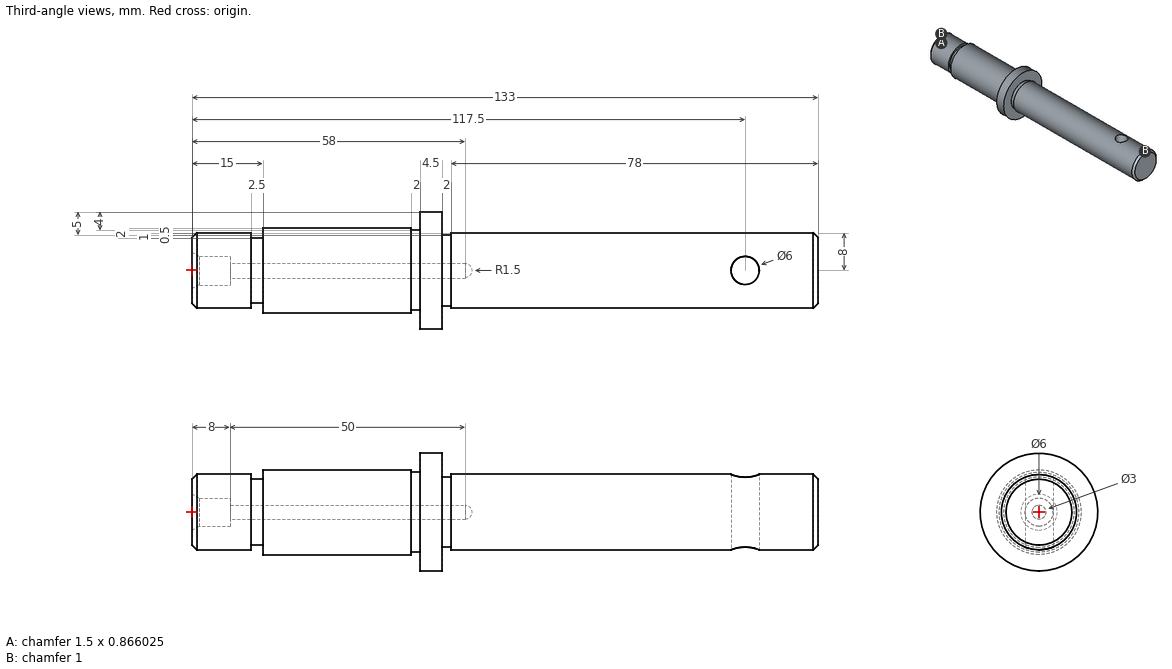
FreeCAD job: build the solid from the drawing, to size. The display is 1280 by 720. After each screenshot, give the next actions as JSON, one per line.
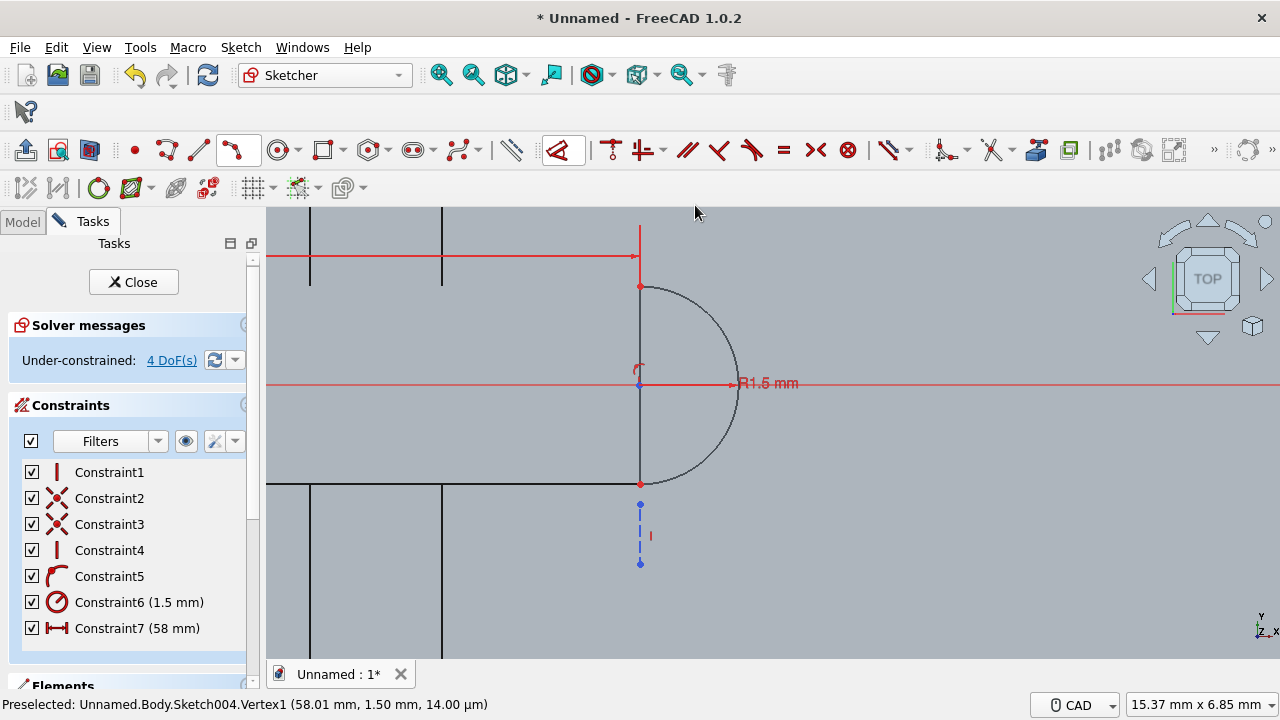
{"action": "left_click", "coordinate": [640, 505]}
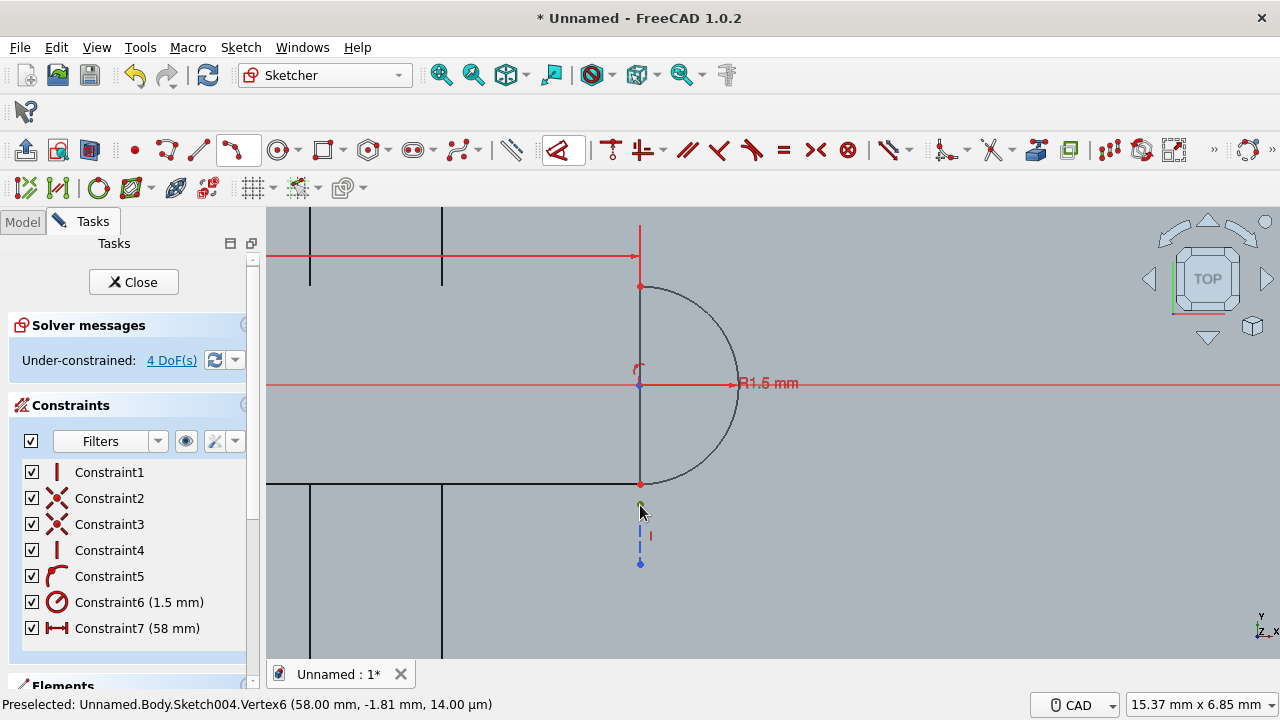
{"action": "left_click", "coordinate": [580, 150]}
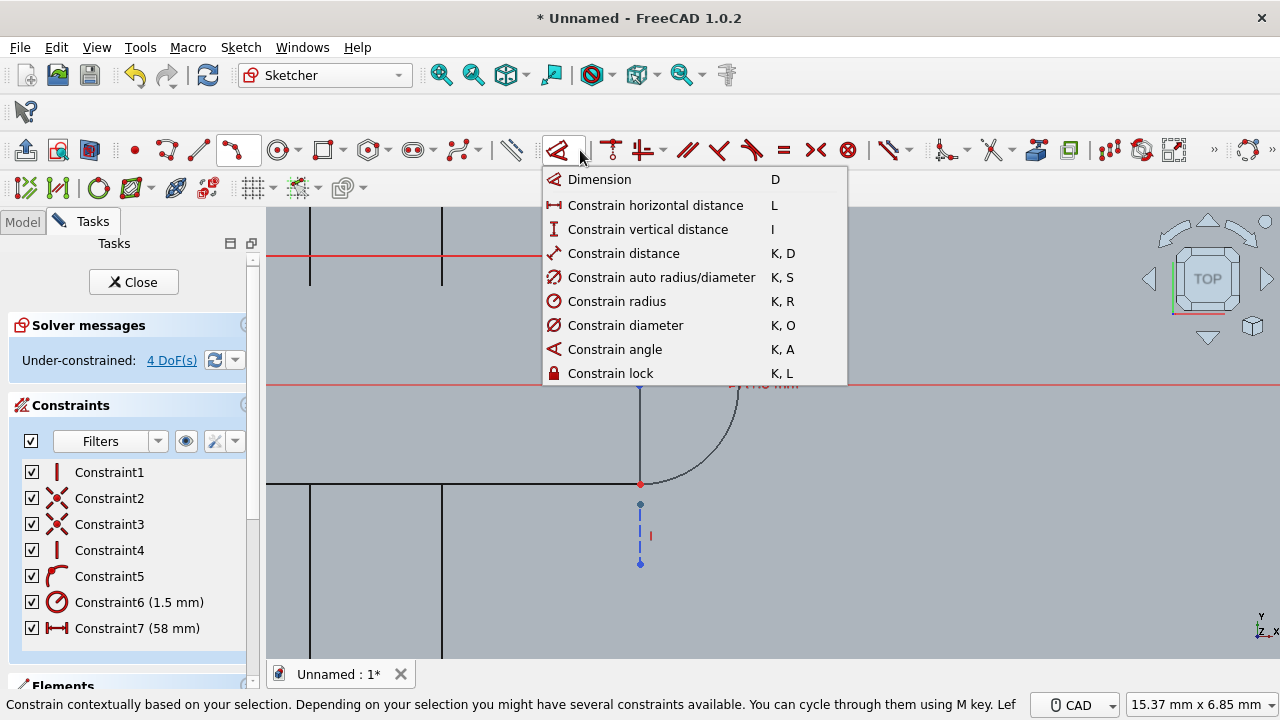
{"action": "left_click", "coordinate": [695, 205]}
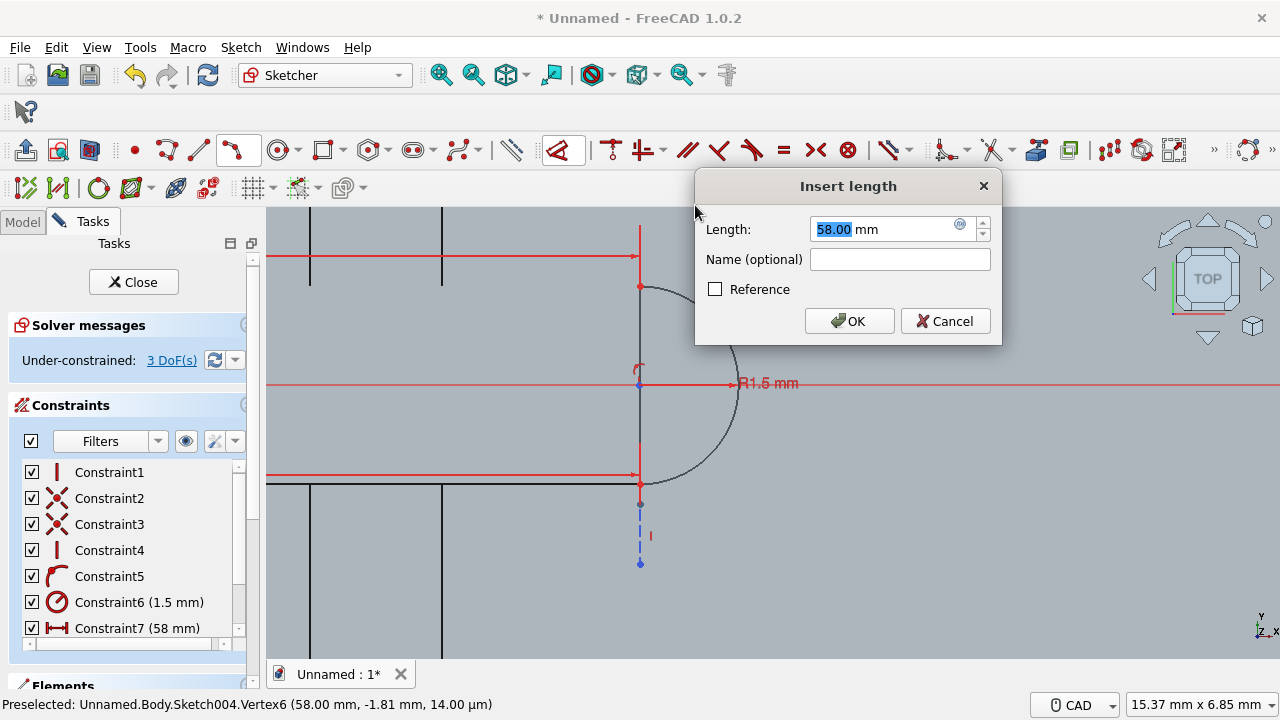
{"action": "type", "text": "58"}
{"action": "key", "text": "Return"}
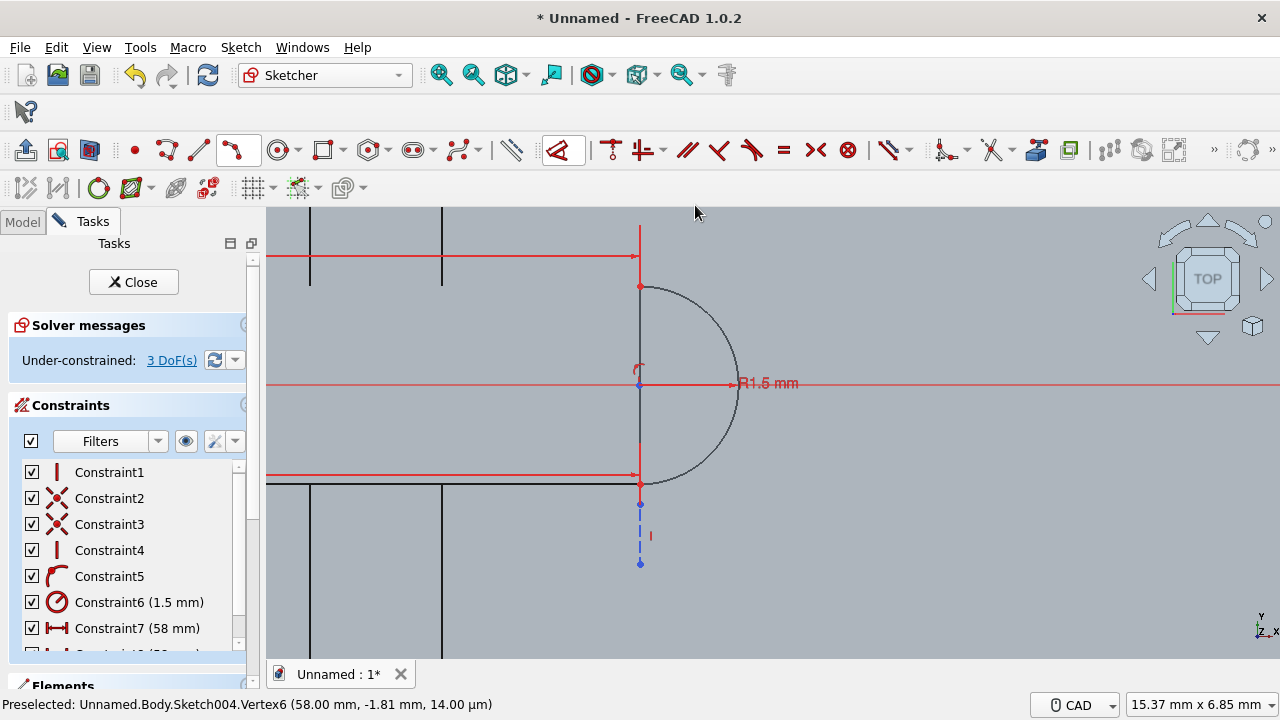
{"action": "left_click", "coordinate": [640, 385]}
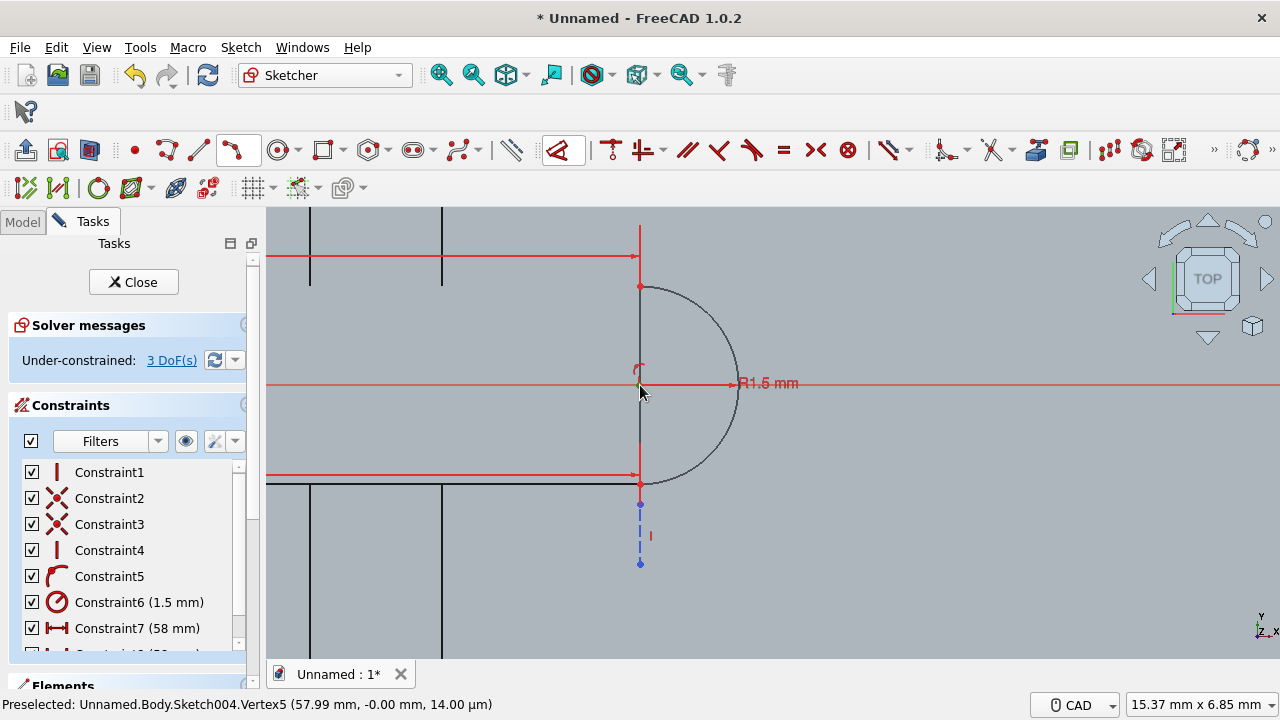
{"action": "left_click", "coordinate": [580, 150]}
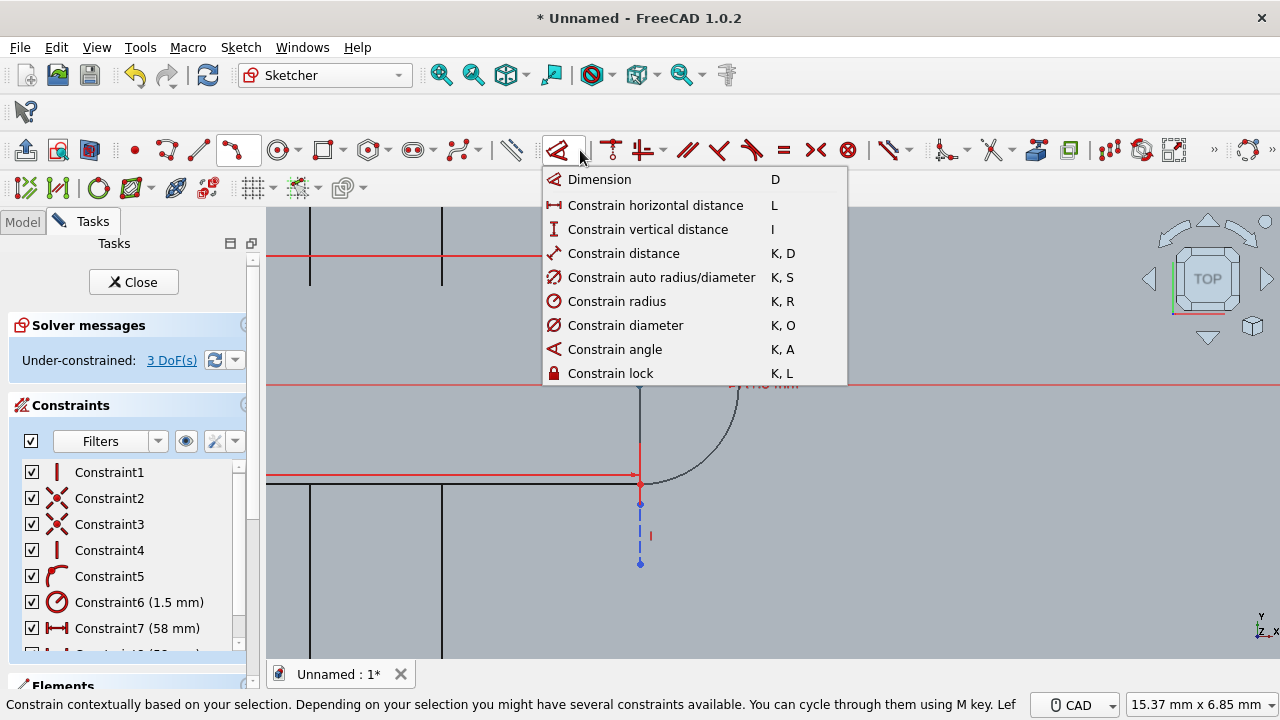
{"action": "left_click", "coordinate": [695, 205]}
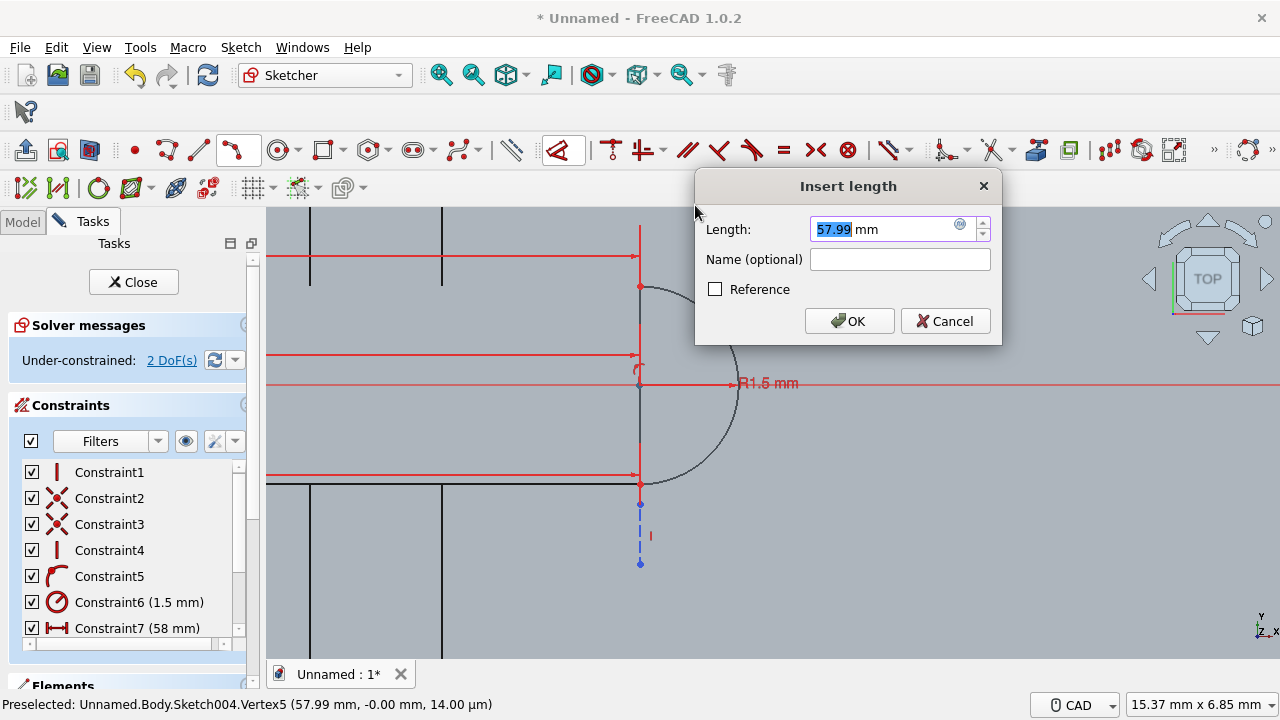
{"action": "type", "text": "58"}
{"action": "key", "text": "Return"}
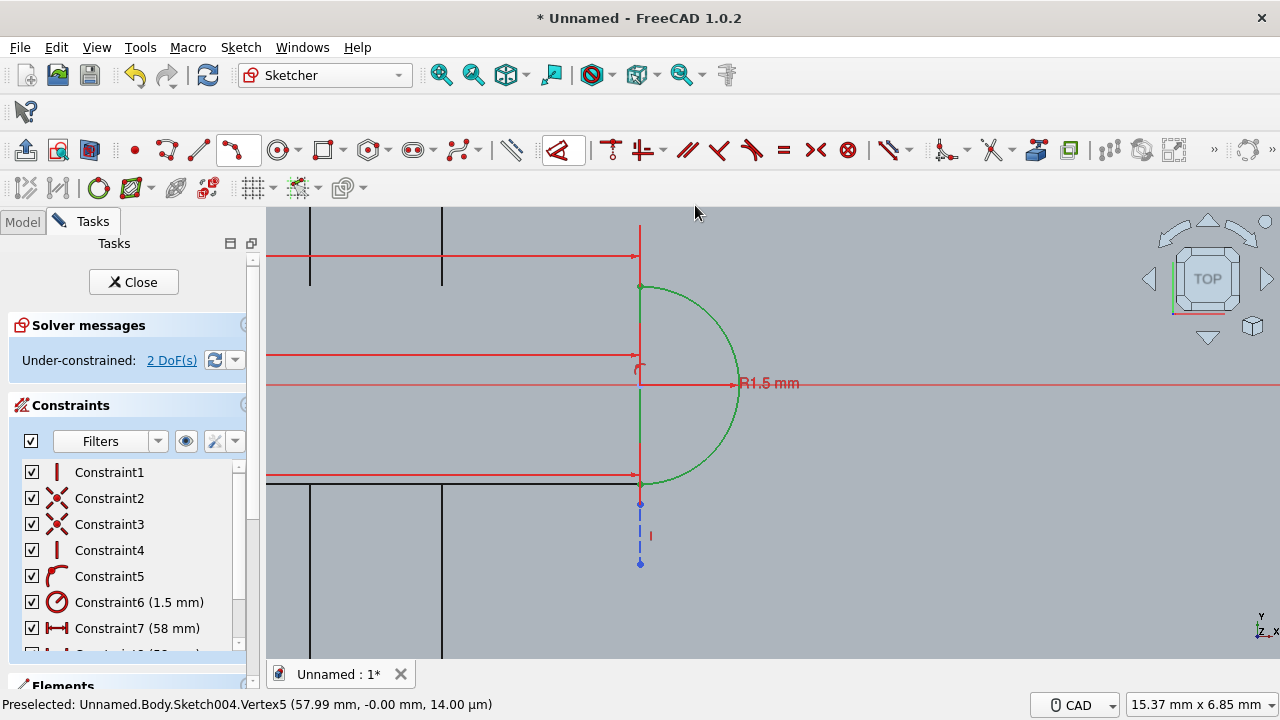
{"action": "left_click", "coordinate": [134, 282]}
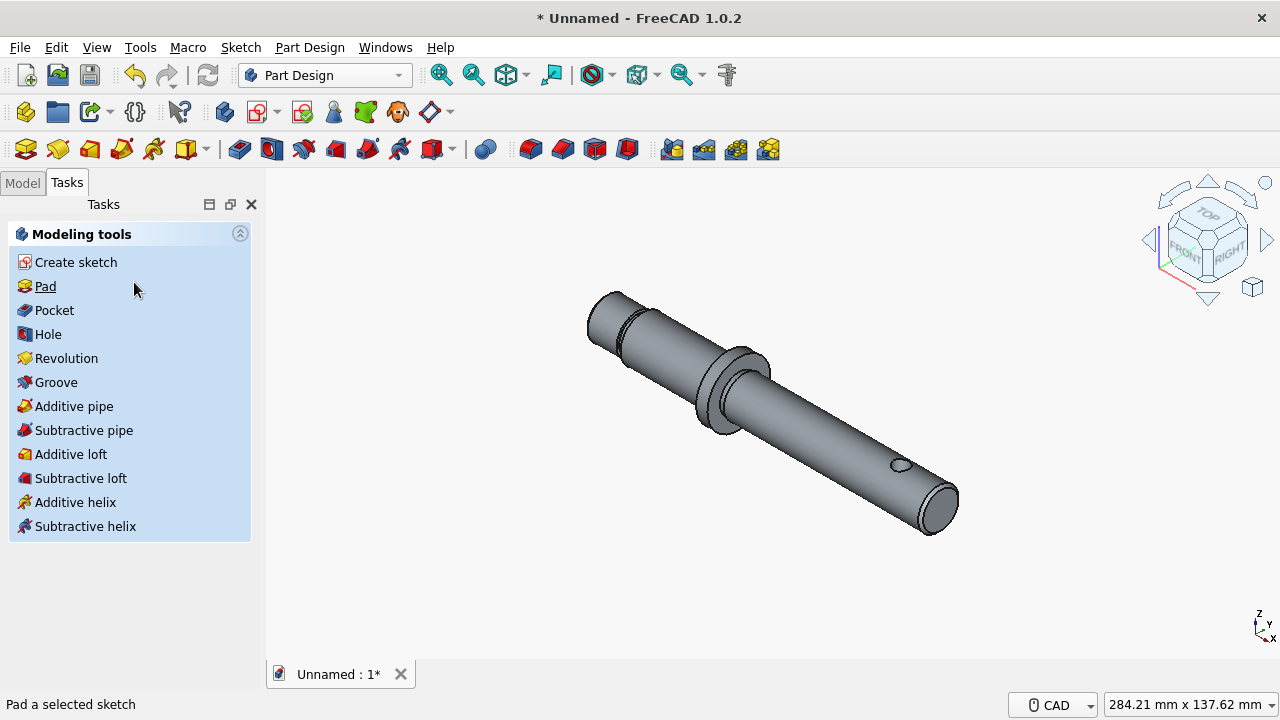
{"action": "left_click", "coordinate": [304, 150]}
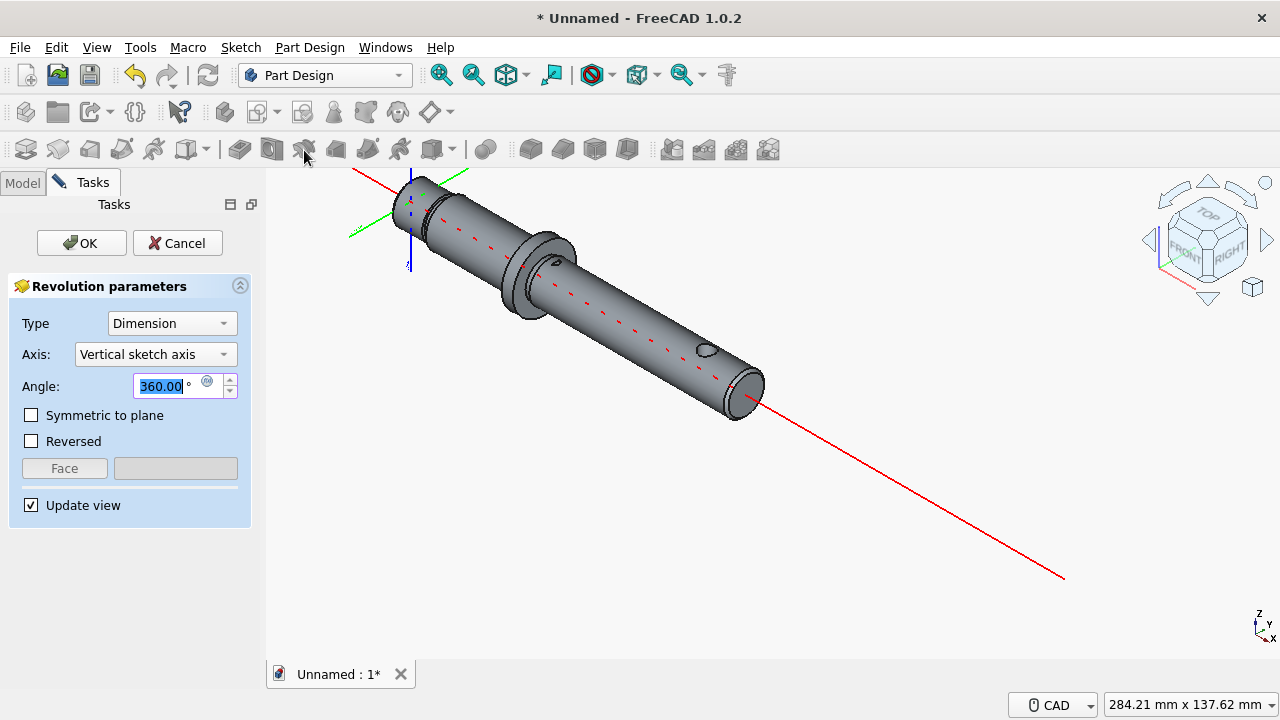
{"action": "left_click", "coordinate": [156, 354]}